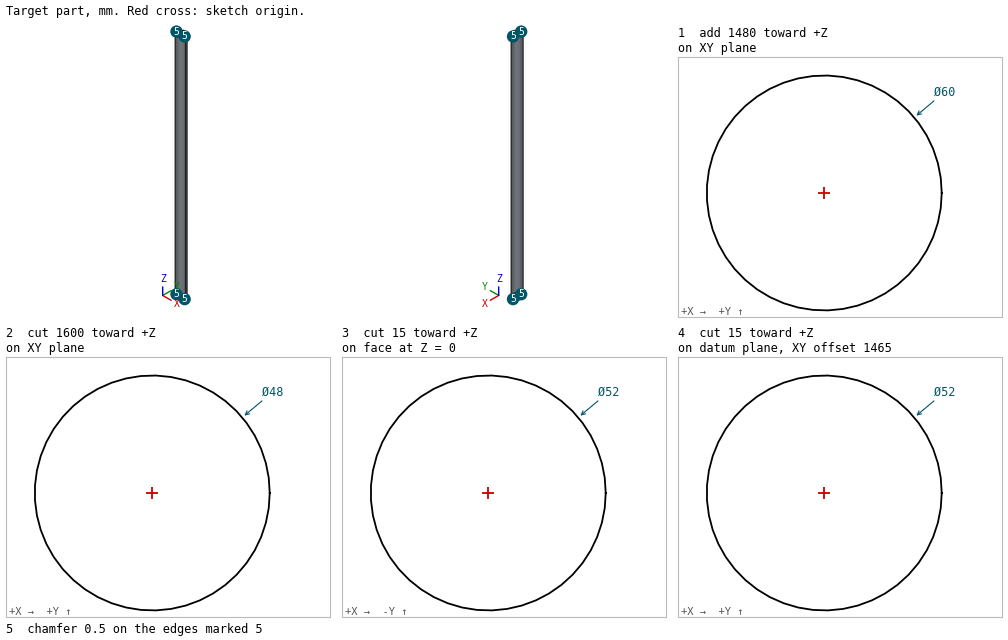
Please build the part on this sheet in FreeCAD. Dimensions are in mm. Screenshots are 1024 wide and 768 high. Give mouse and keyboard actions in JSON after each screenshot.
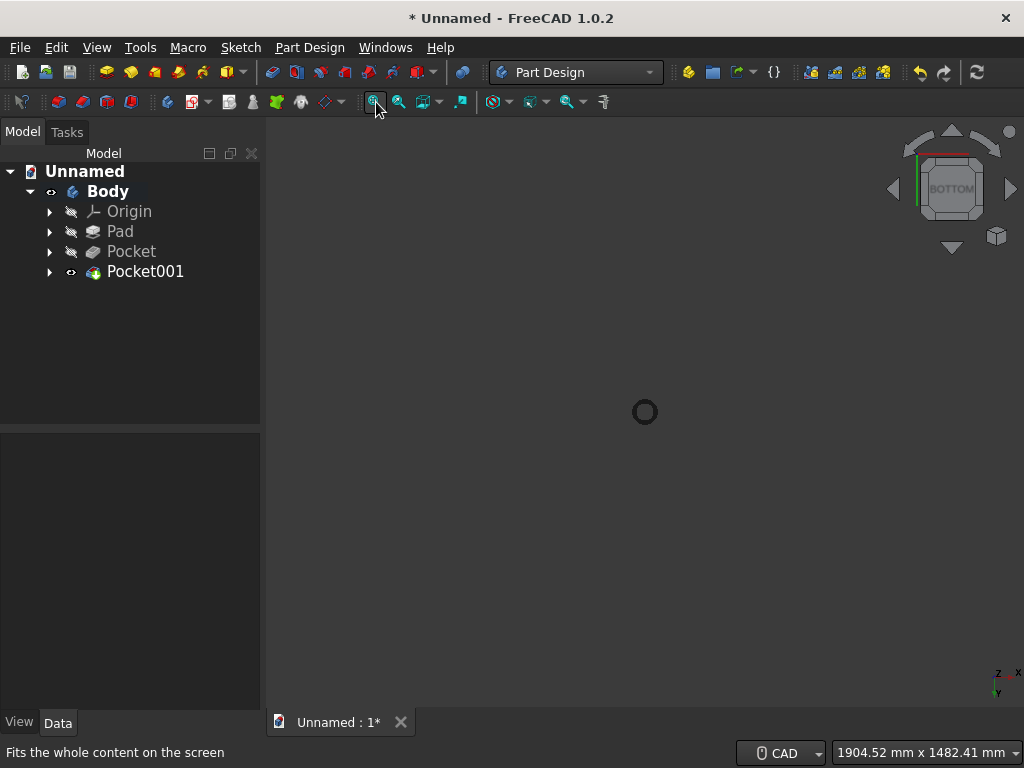
{"action": "left_click", "coordinate": [50, 212]}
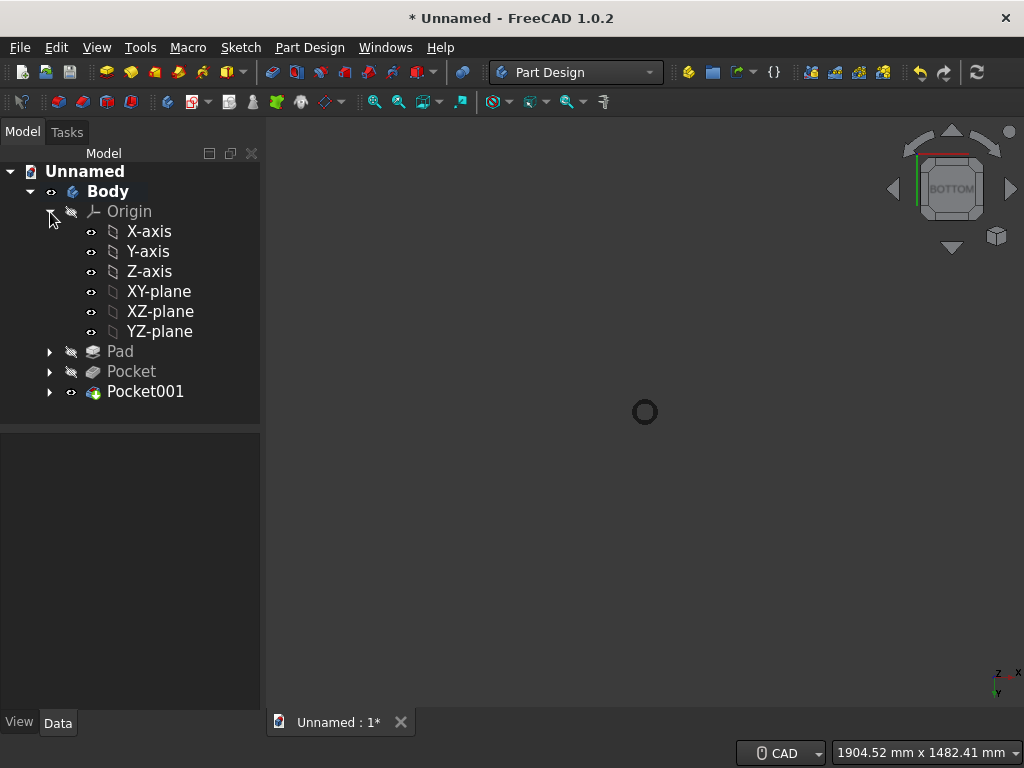
{"action": "left_click", "coordinate": [136, 292]}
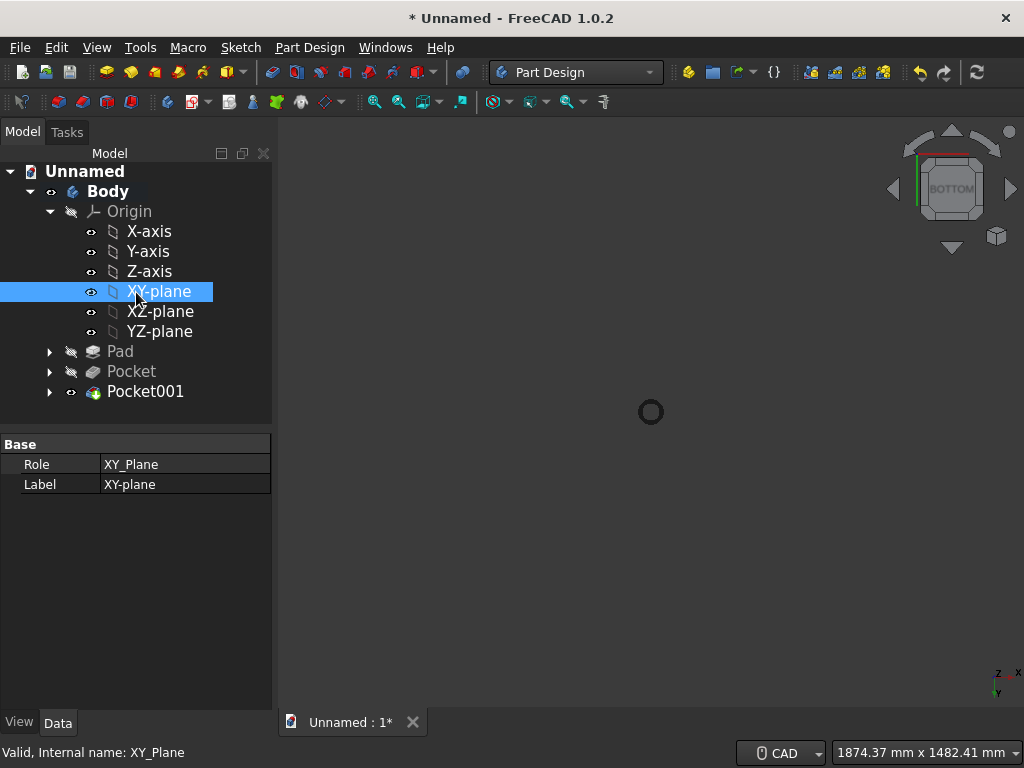
{"action": "left_click", "coordinate": [326, 102]}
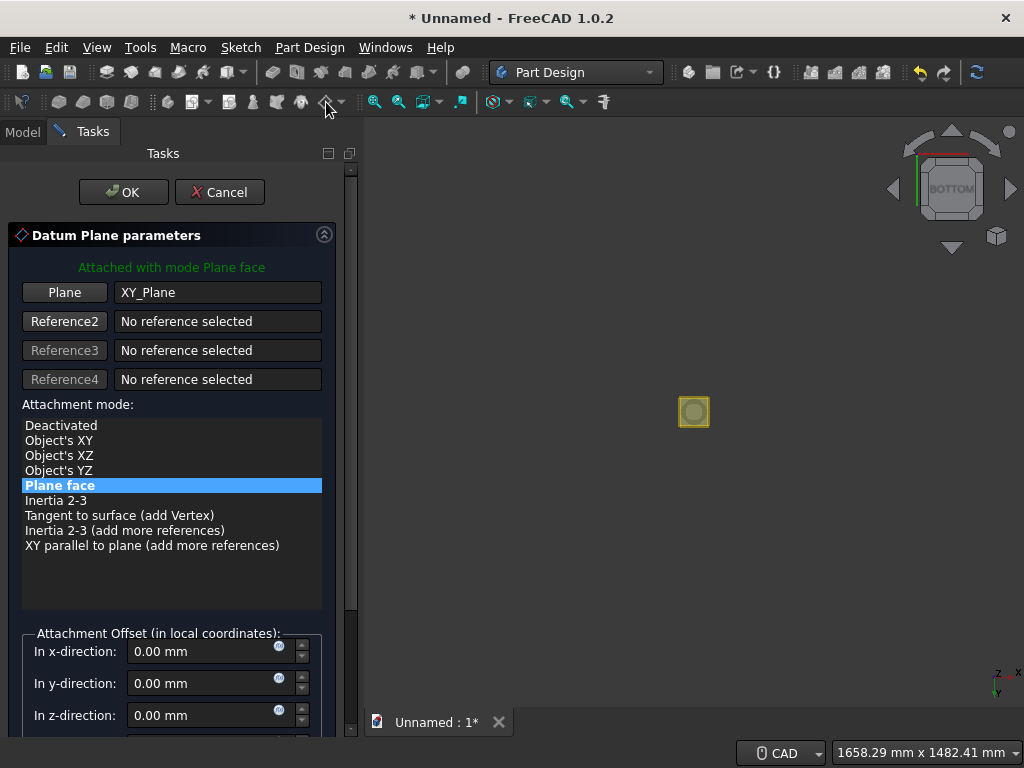
{"action": "triple_click", "coordinate": [210, 715]}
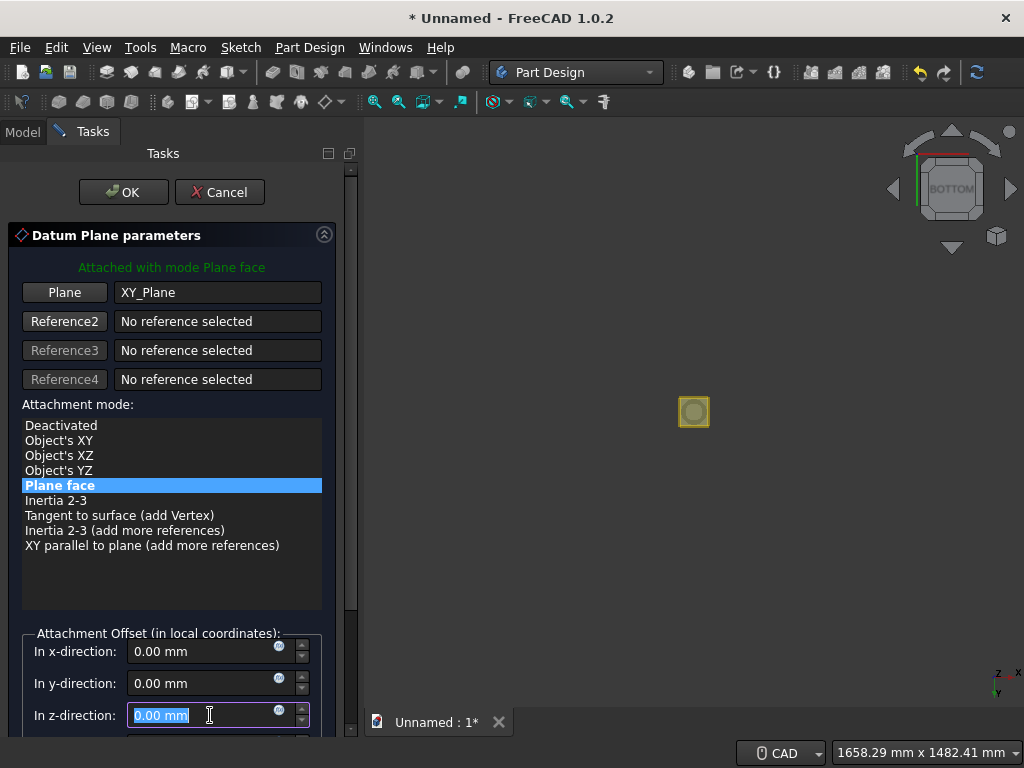
{"action": "type", "text": "1465"}
{"action": "key", "text": "Tab"}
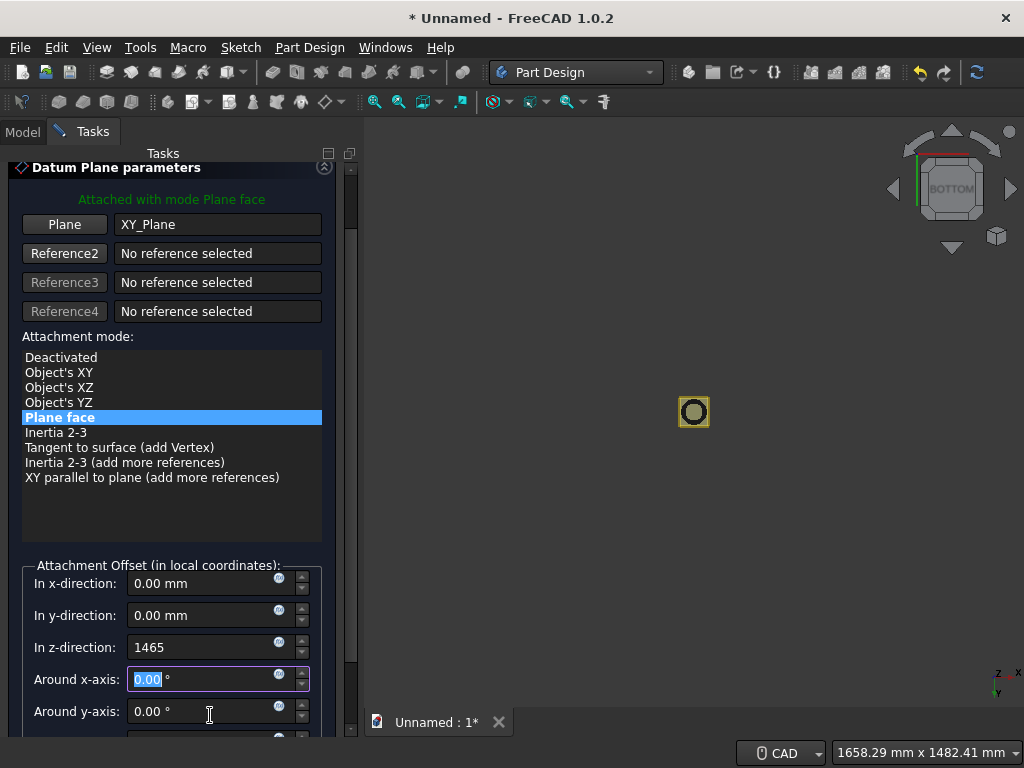
{"action": "scroll", "coordinate": [351, 450], "scroll_direction": "up", "scroll_amount": 2}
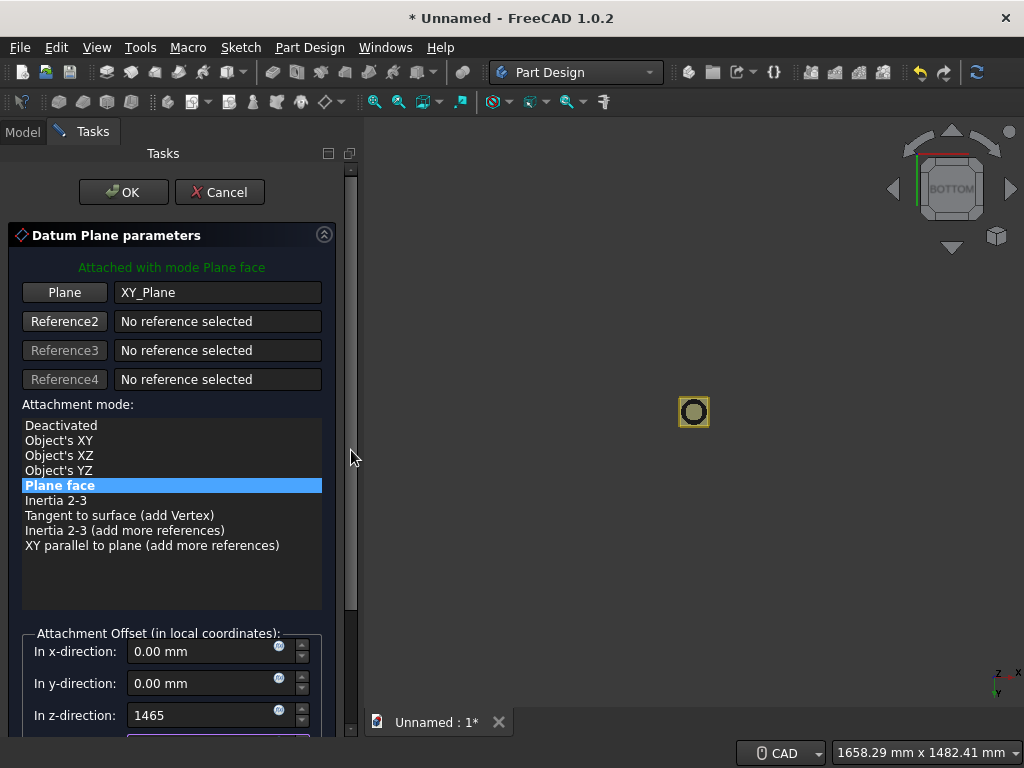
{"action": "left_click", "coordinate": [124, 192]}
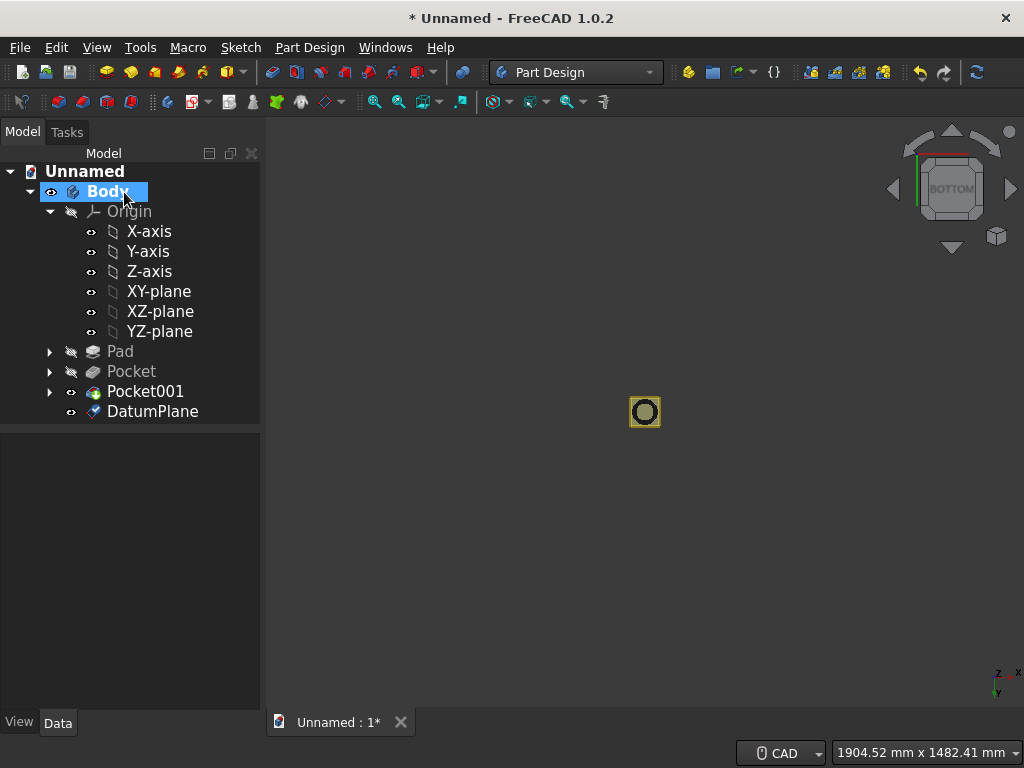
{"action": "left_click", "coordinate": [116, 412]}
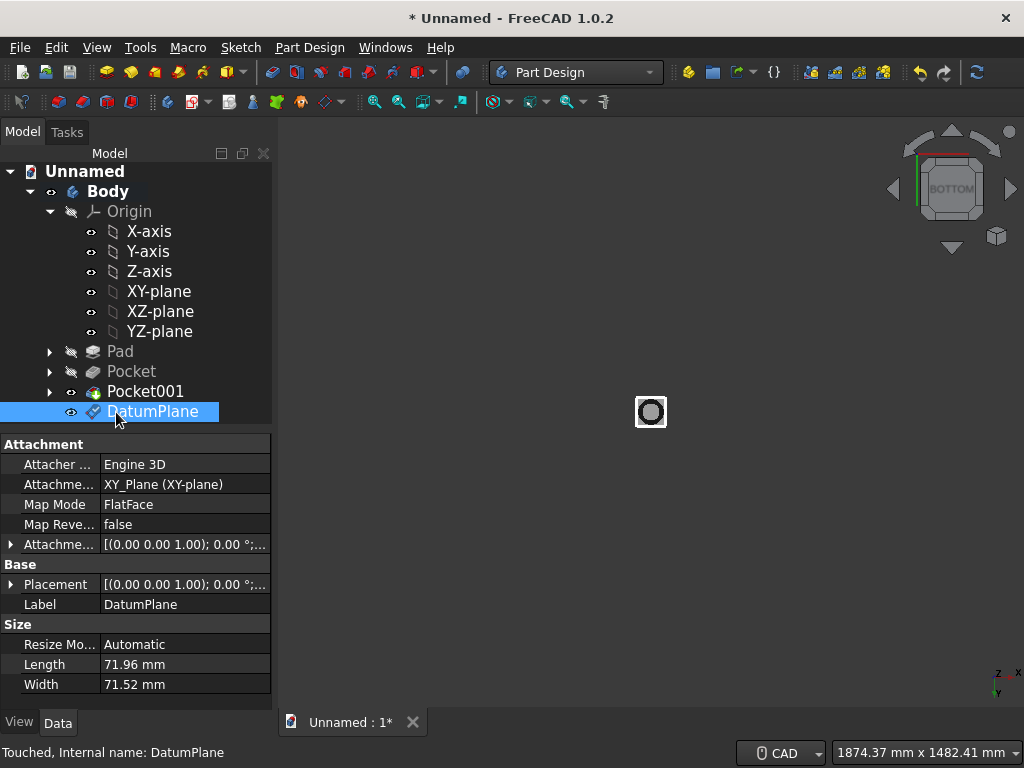
{"action": "left_click", "coordinate": [192, 102]}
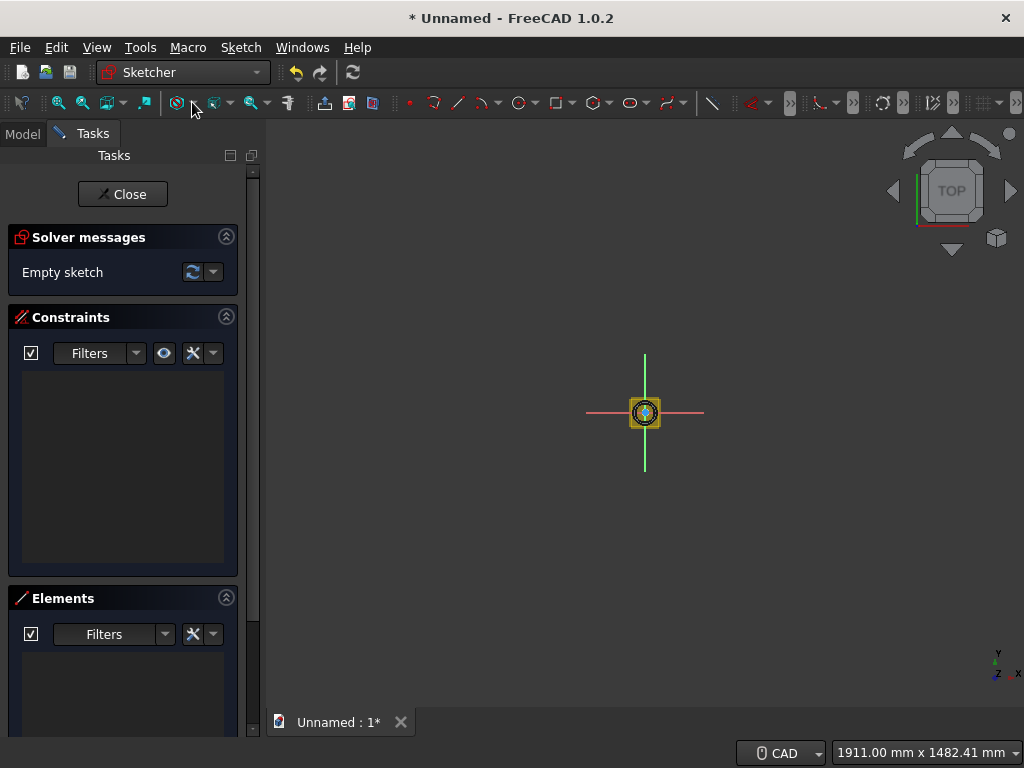
{"action": "left_click", "coordinate": [374, 104]}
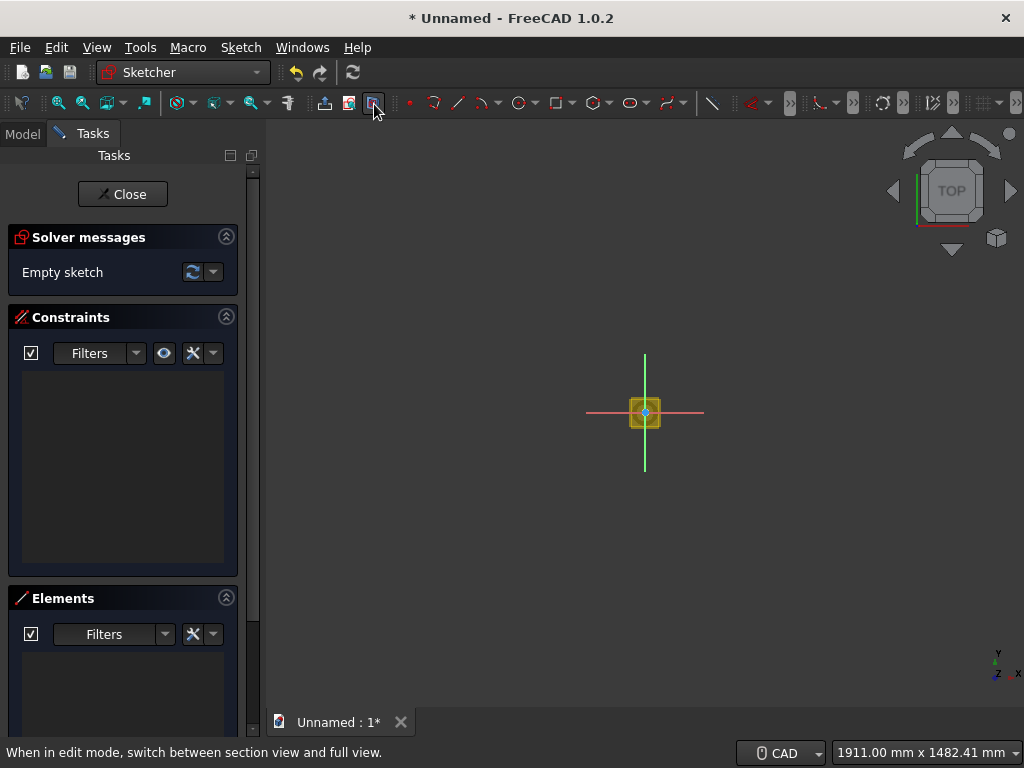
{"action": "scroll", "coordinate": [649, 413], "scroll_direction": "up", "scroll_amount": 15}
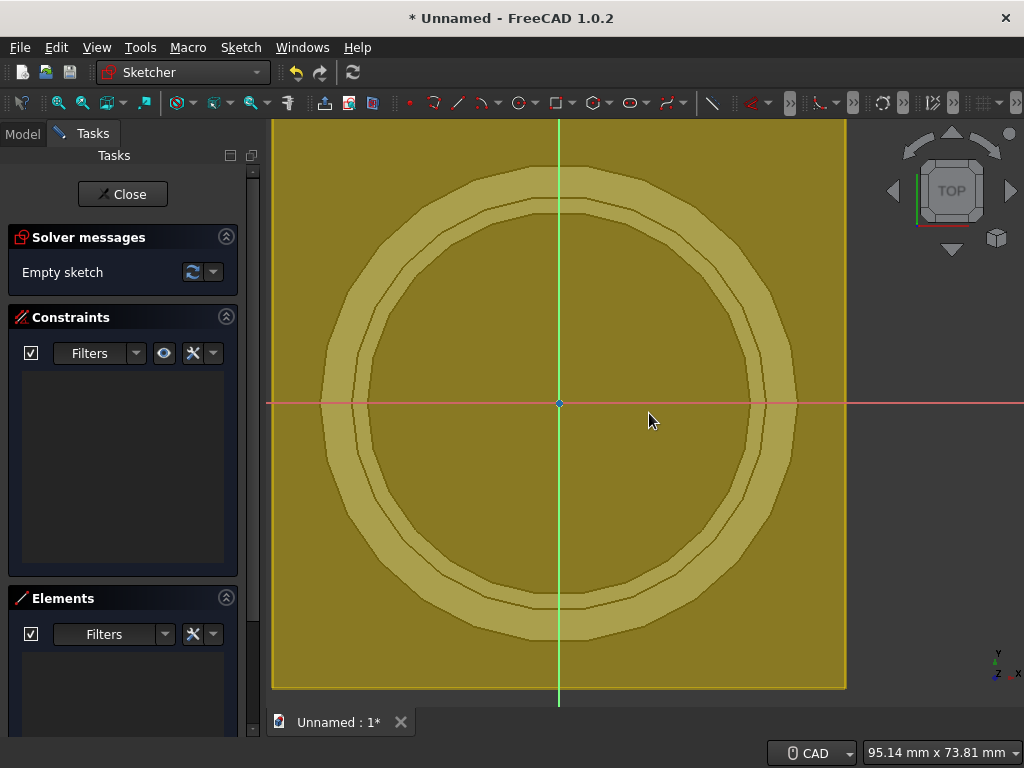
{"action": "left_click", "coordinate": [520, 104]}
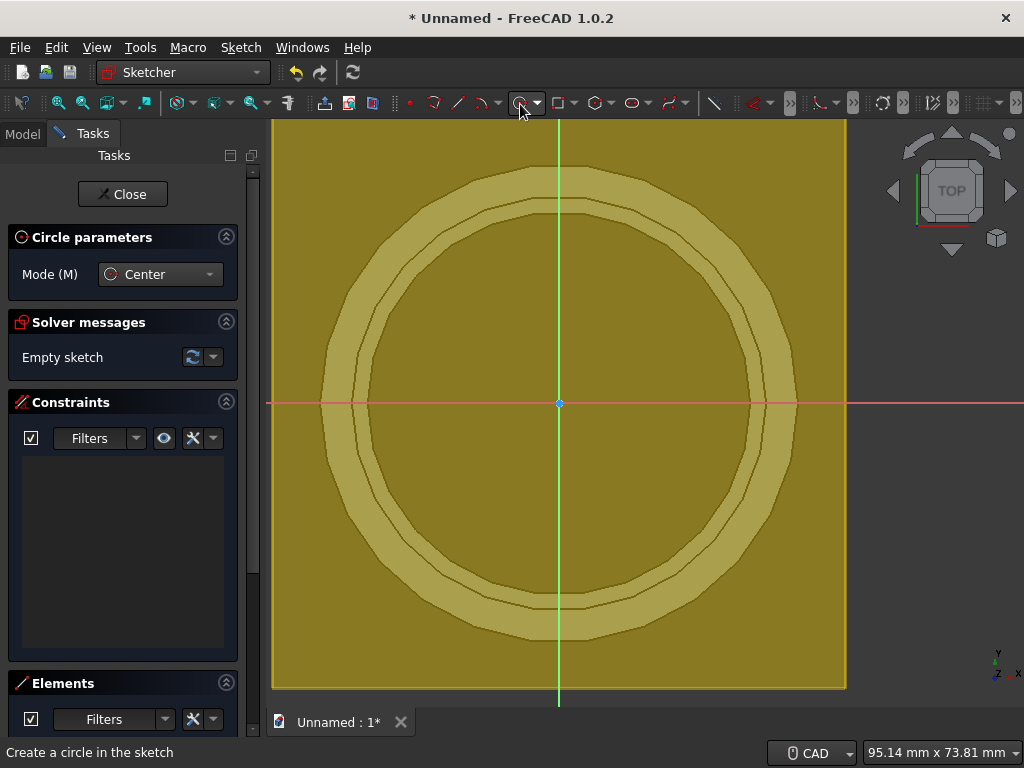
{"action": "left_click", "coordinate": [559, 403]}
{"action": "mouse_move", "coordinate": [705, 257]}